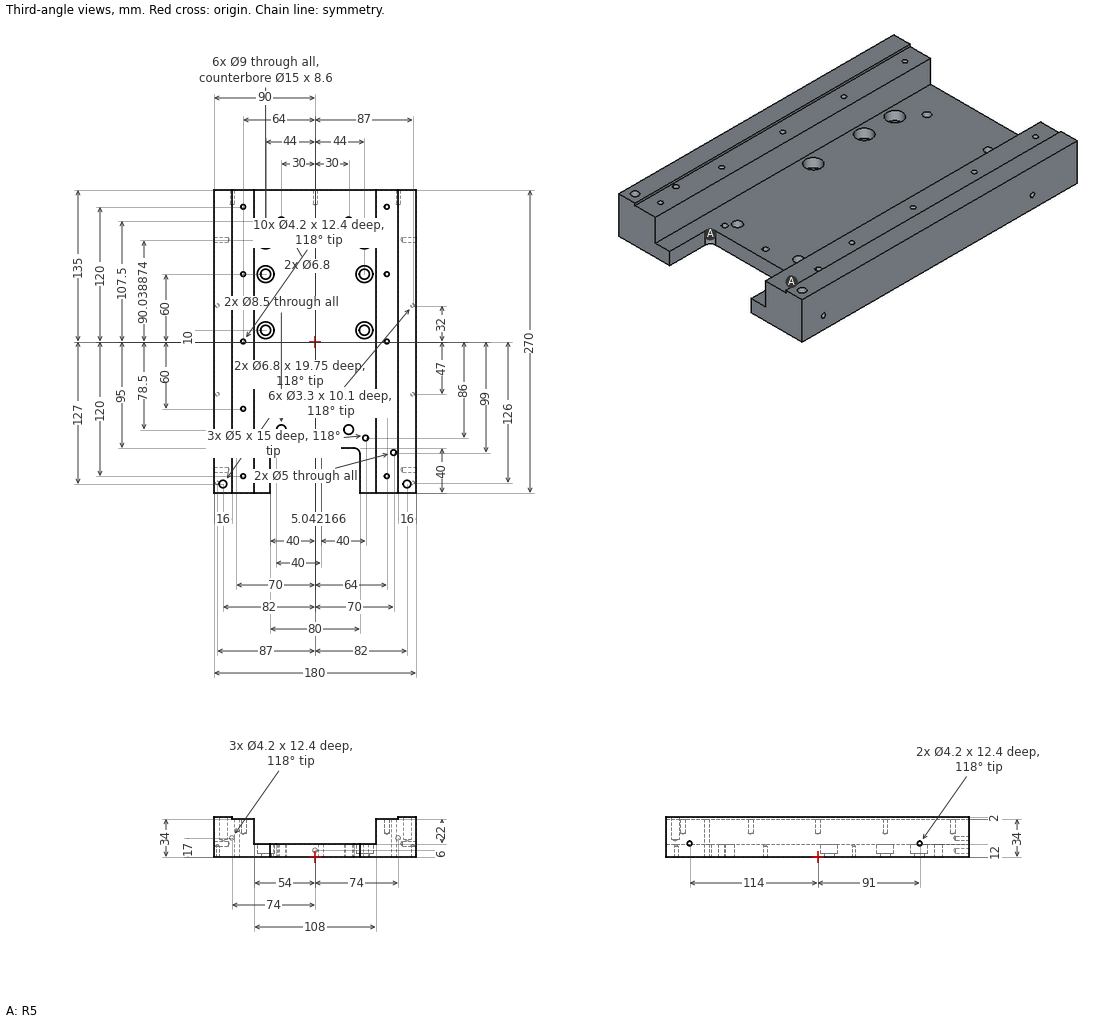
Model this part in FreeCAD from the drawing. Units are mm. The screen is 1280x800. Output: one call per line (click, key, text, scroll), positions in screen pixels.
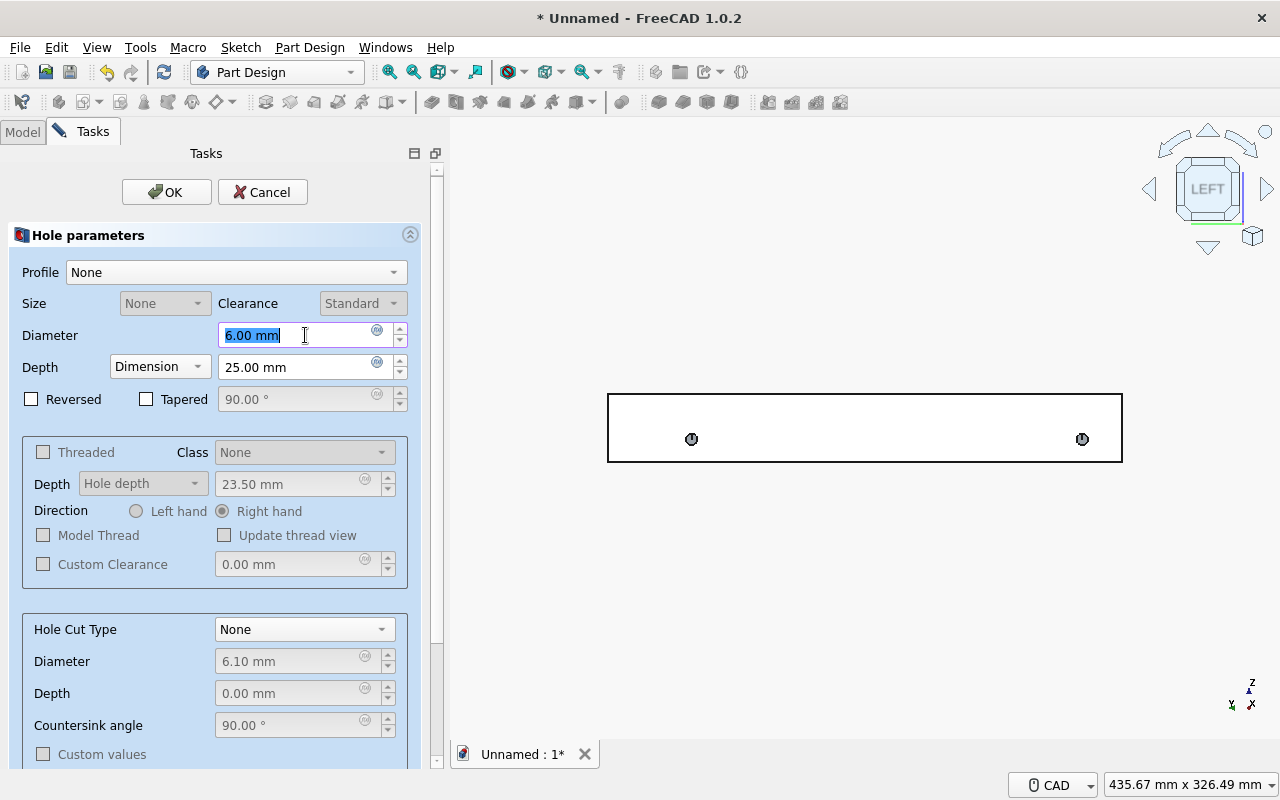
text(4.2)
key(Tab)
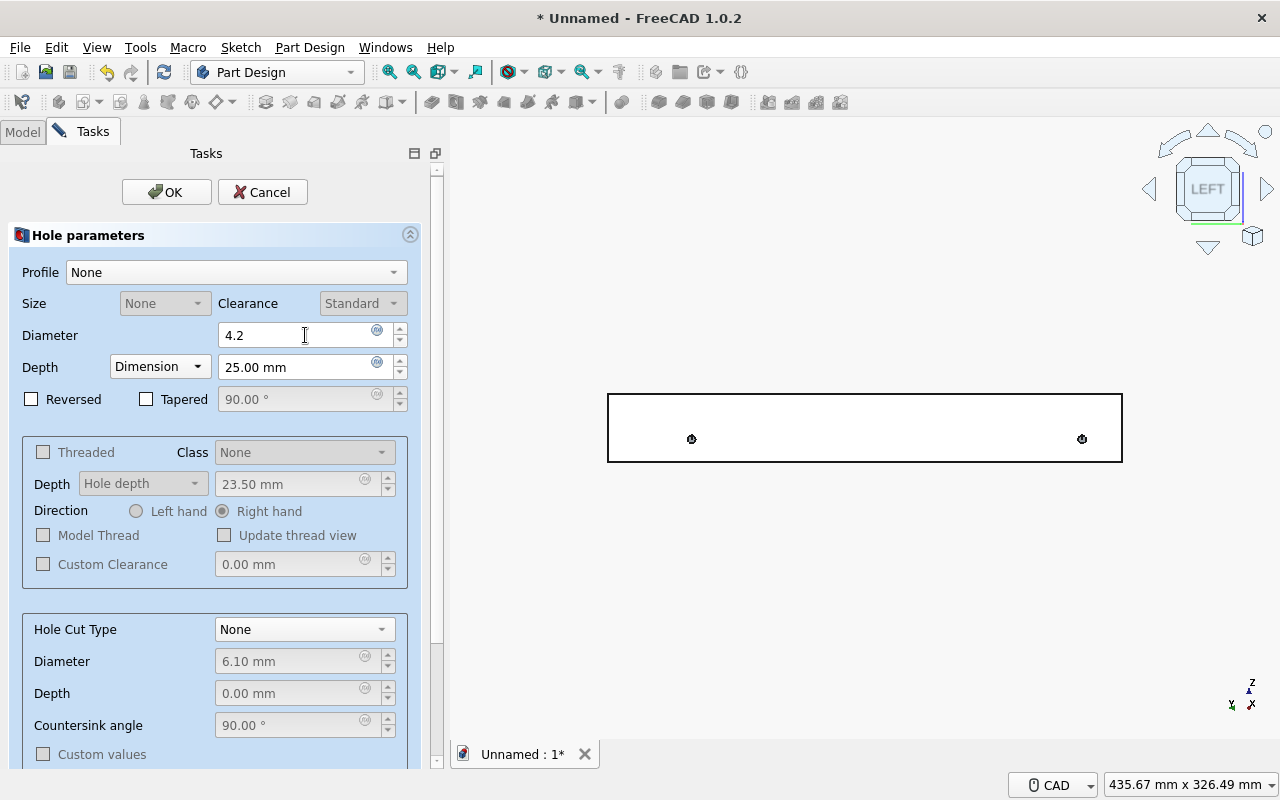
triple_click(305, 367)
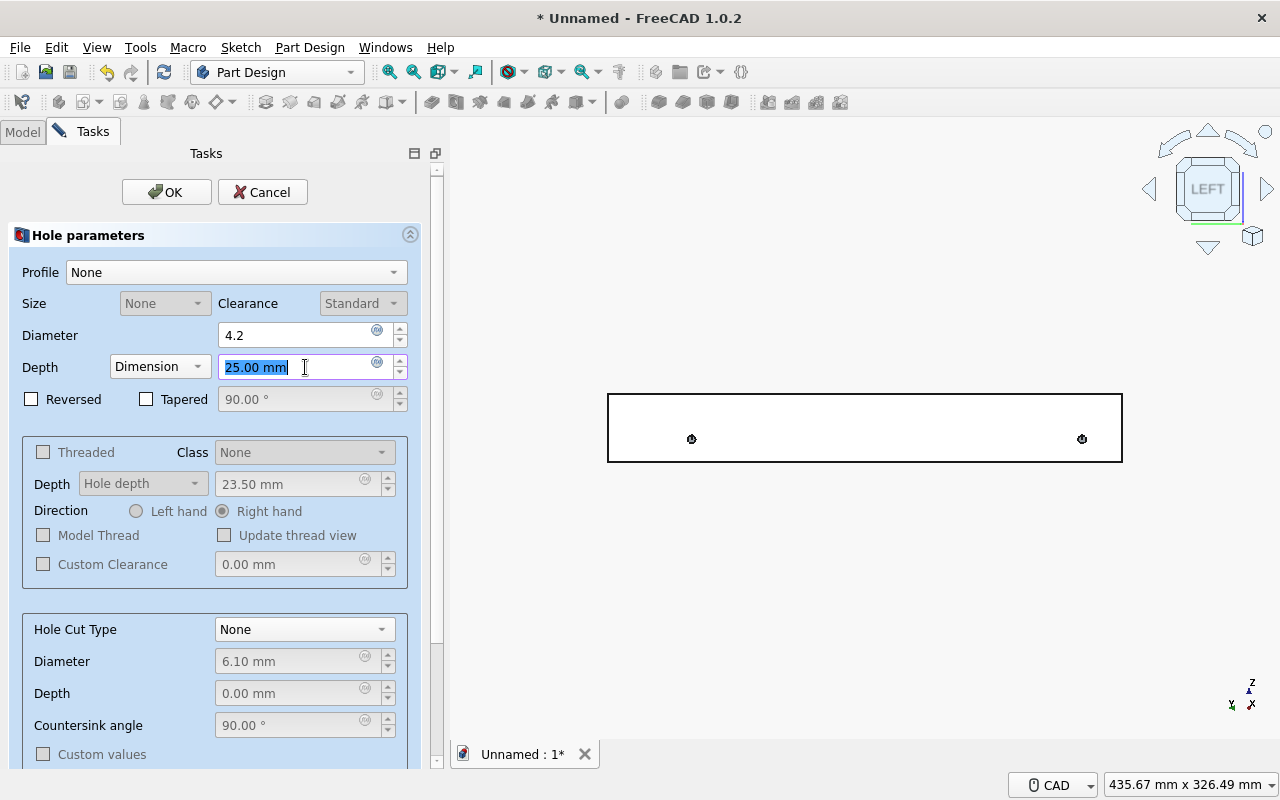
text(12.4)
key(Tab)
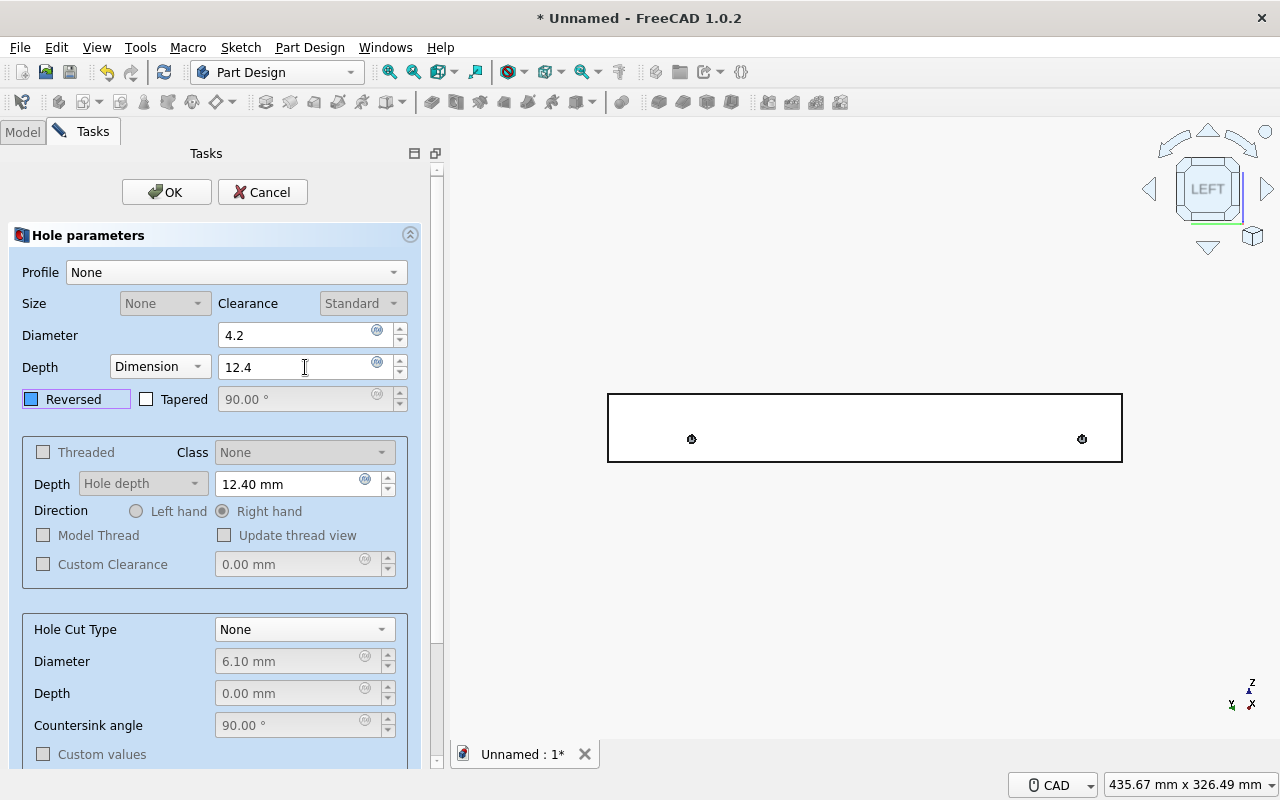
click(167, 192)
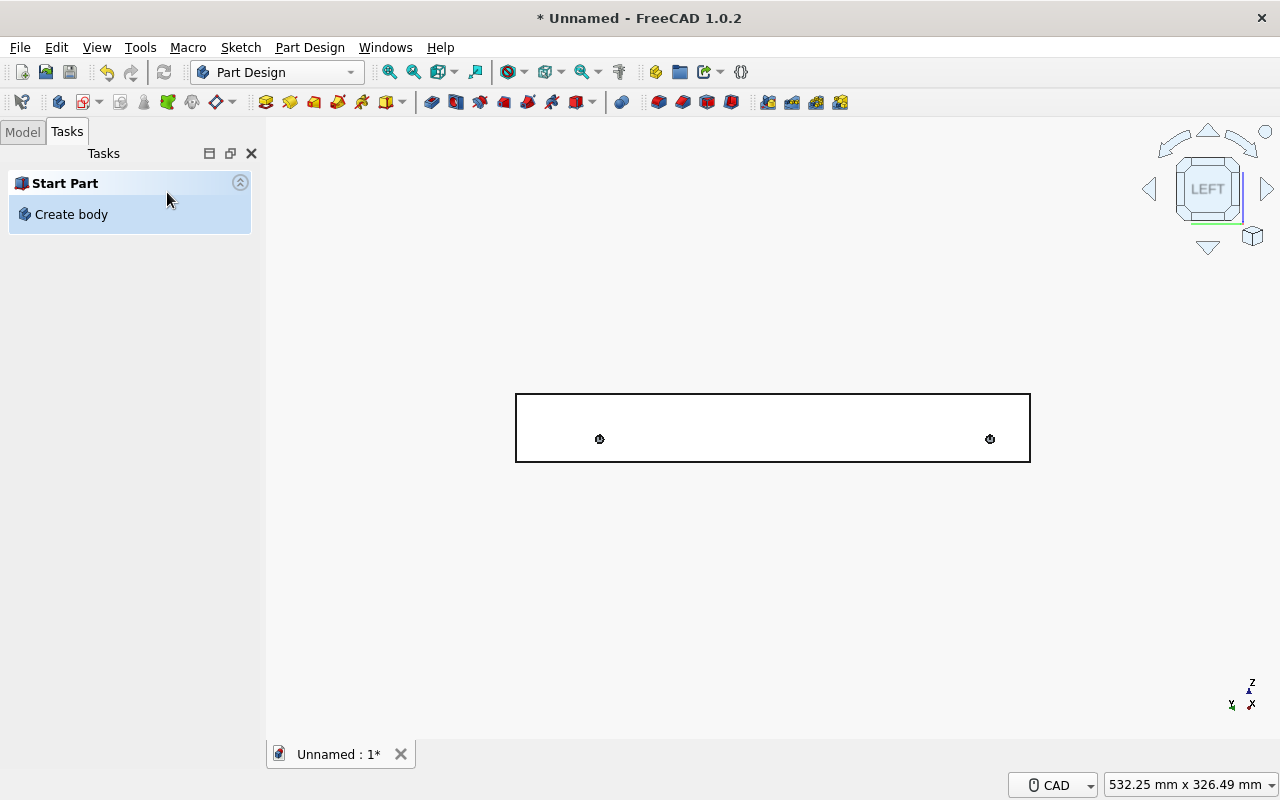
key(0)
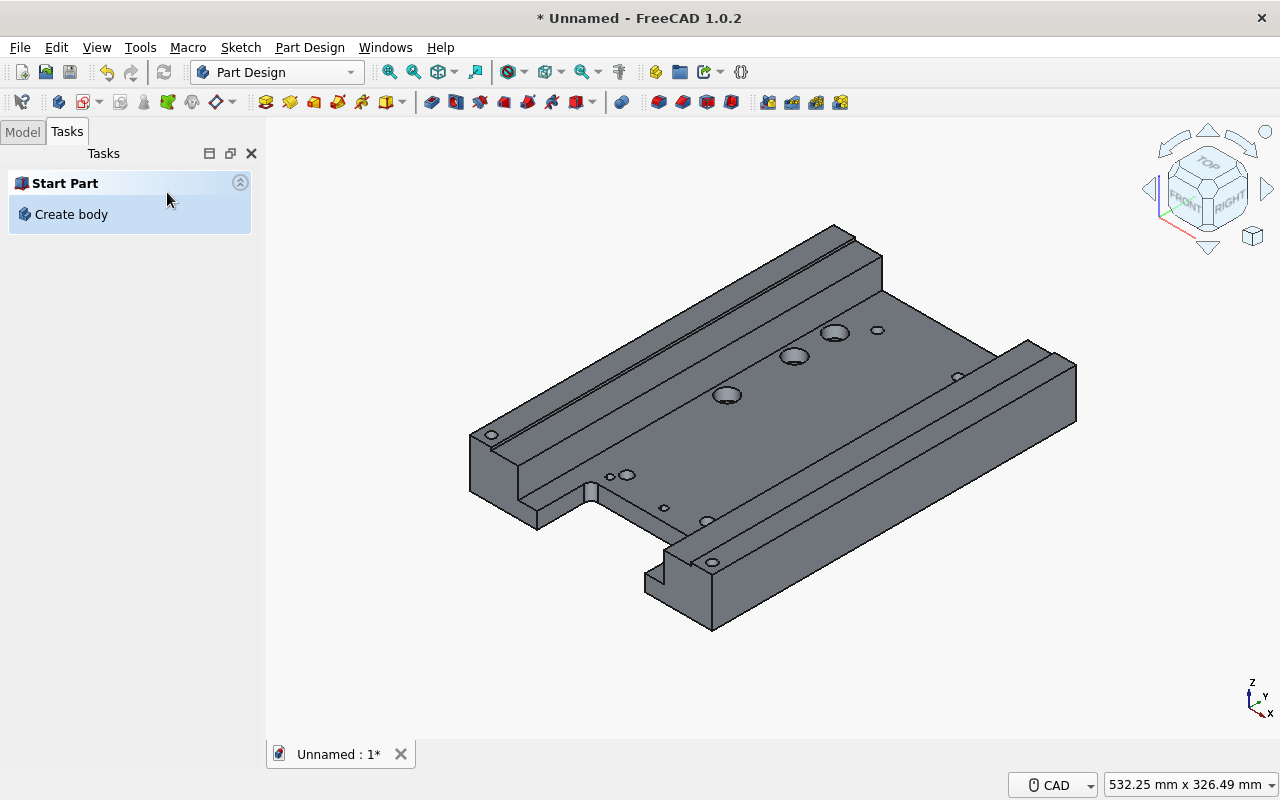
click(1050, 407)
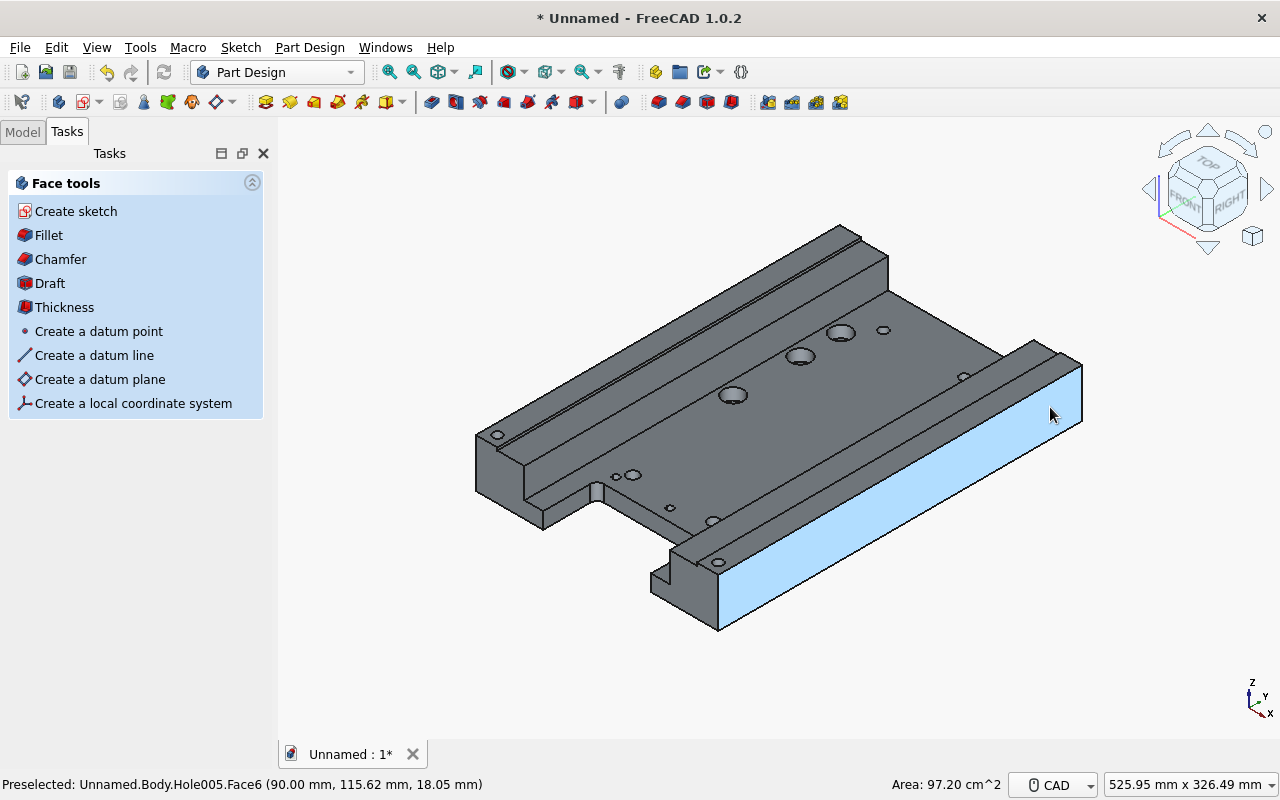
click(84, 102)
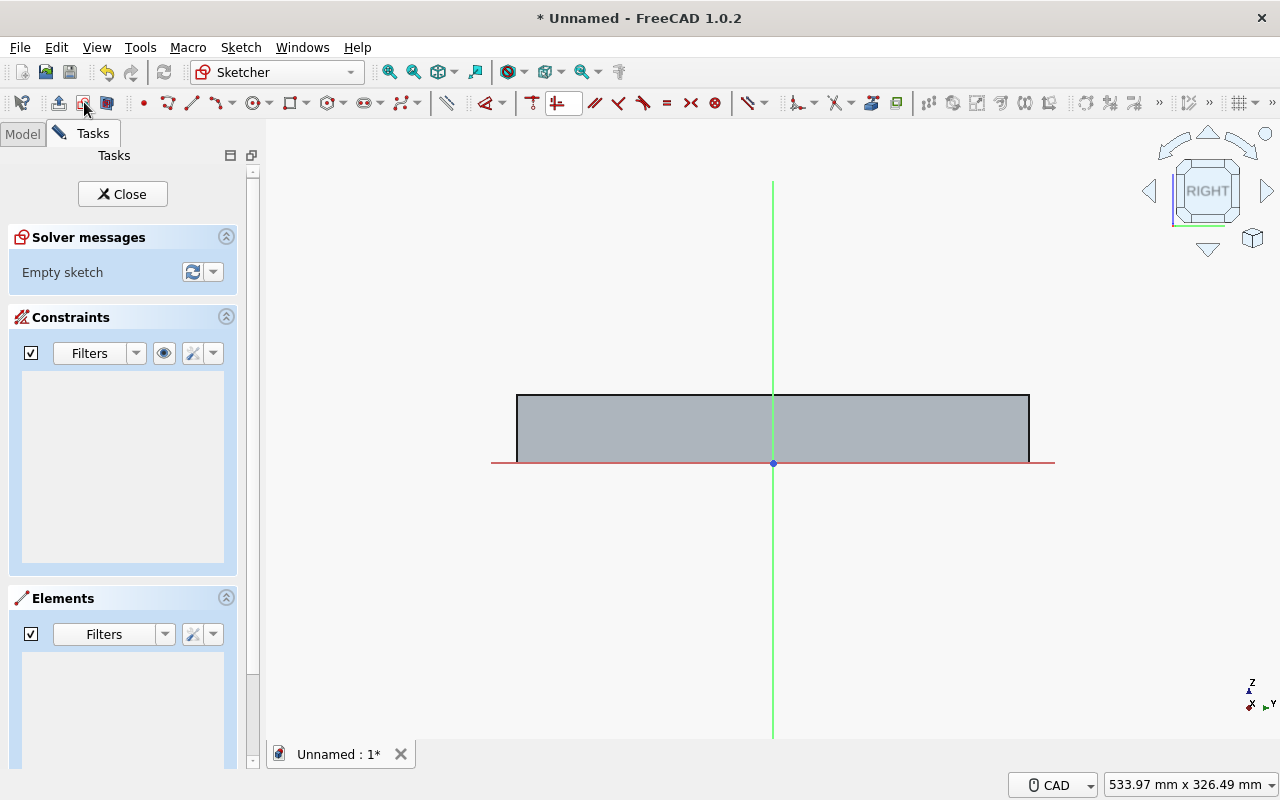
scroll(846, 492, up, 2)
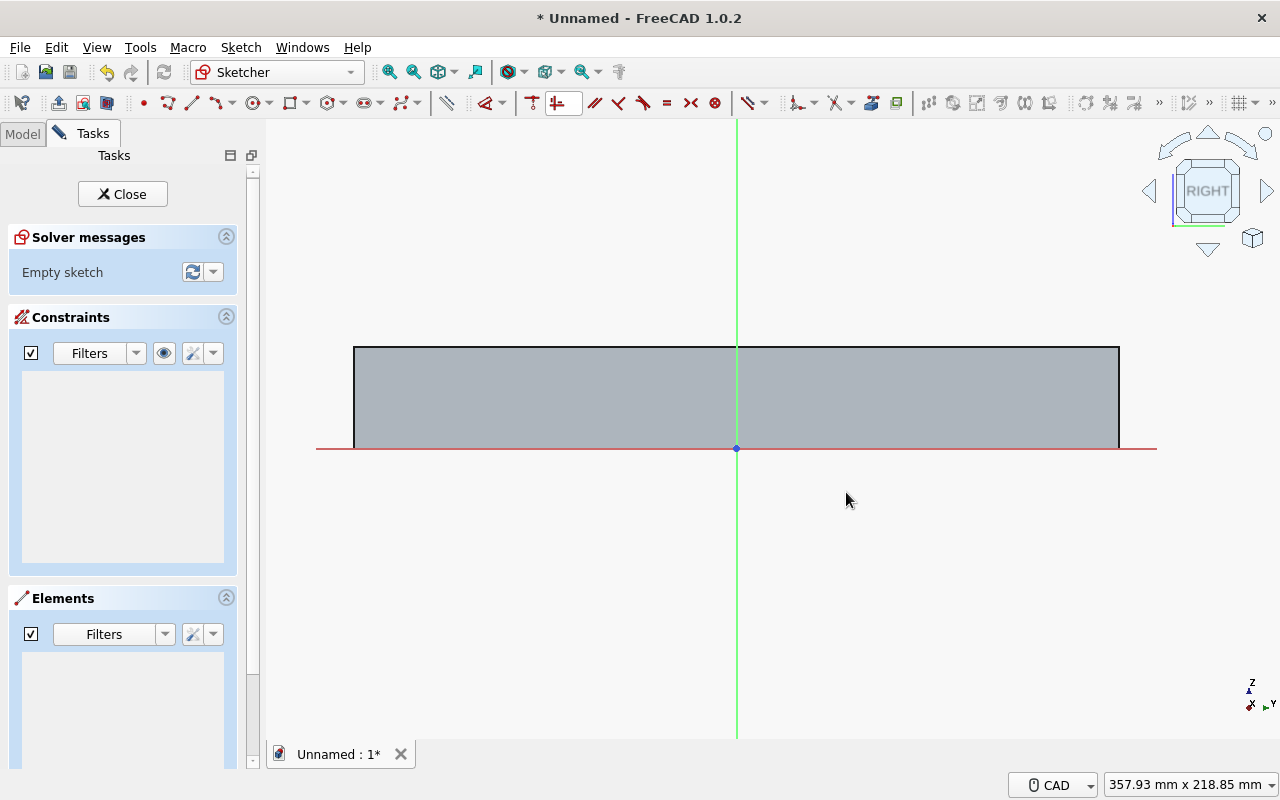
click(254, 104)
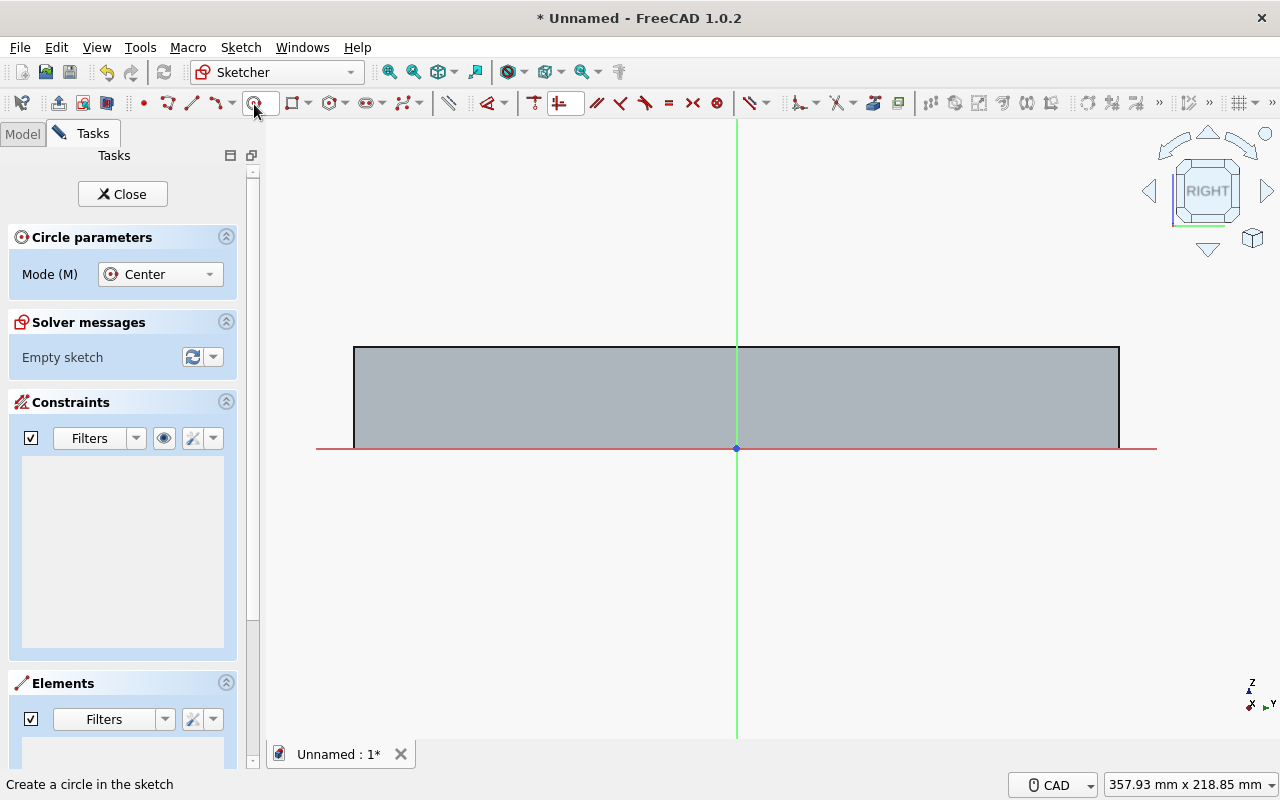
scroll(995, 415, up, 7)